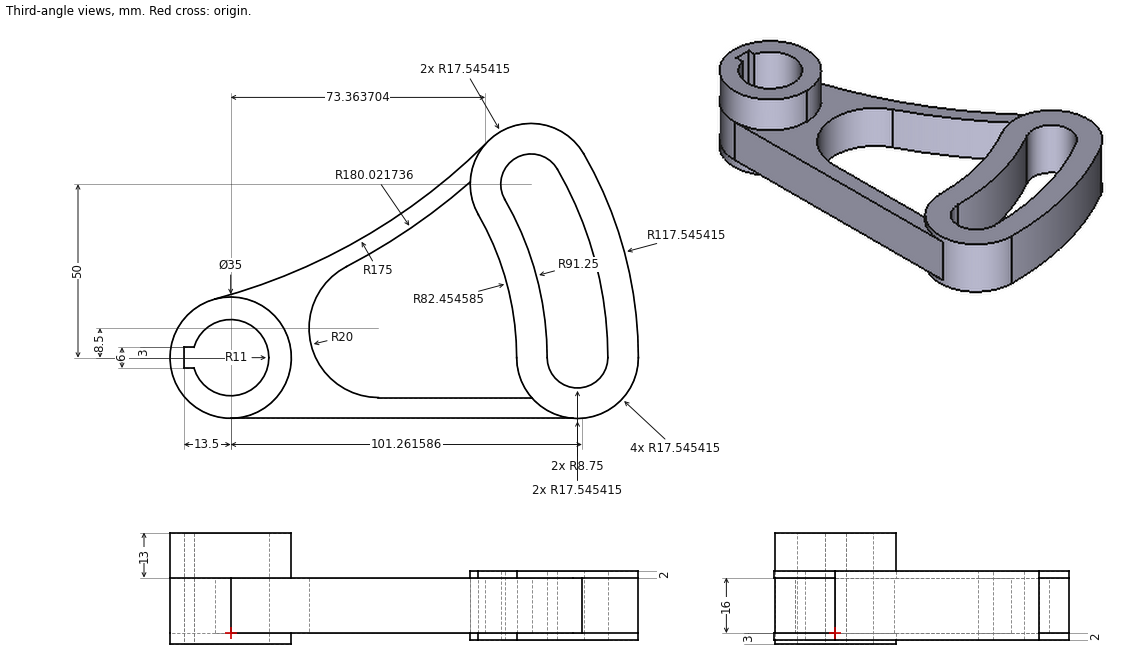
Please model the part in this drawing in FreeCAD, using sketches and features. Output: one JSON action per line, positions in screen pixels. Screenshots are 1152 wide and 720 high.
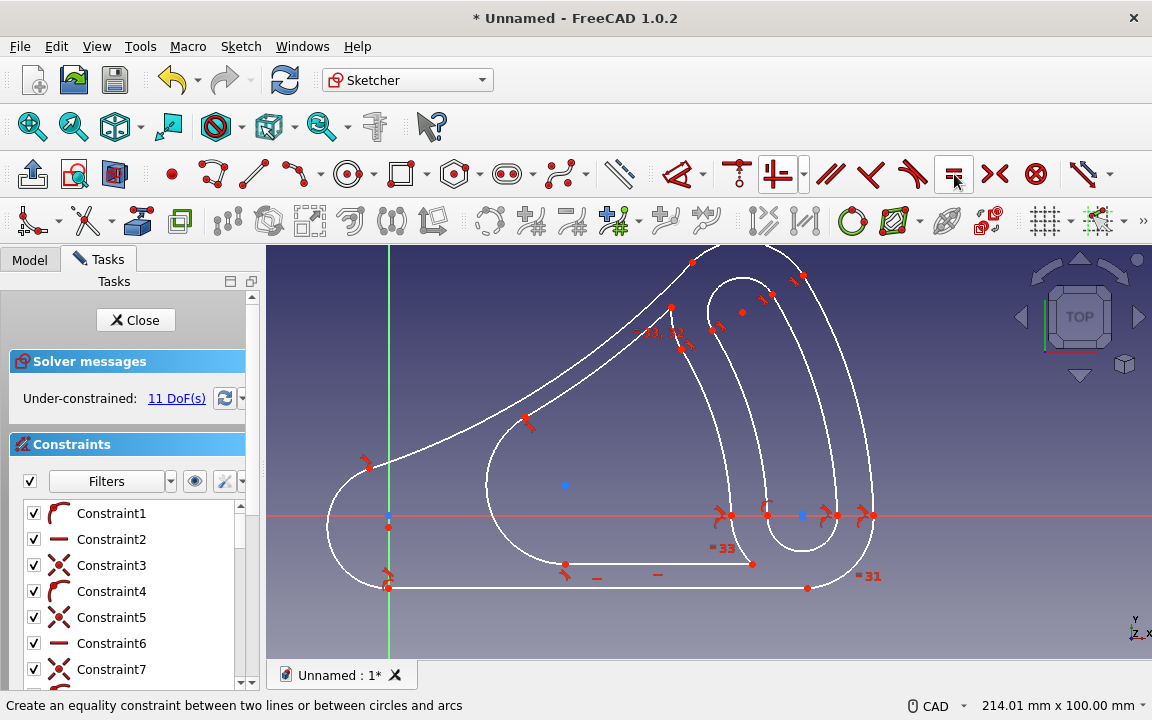
{"action": "left_click", "coordinate": [389, 527]}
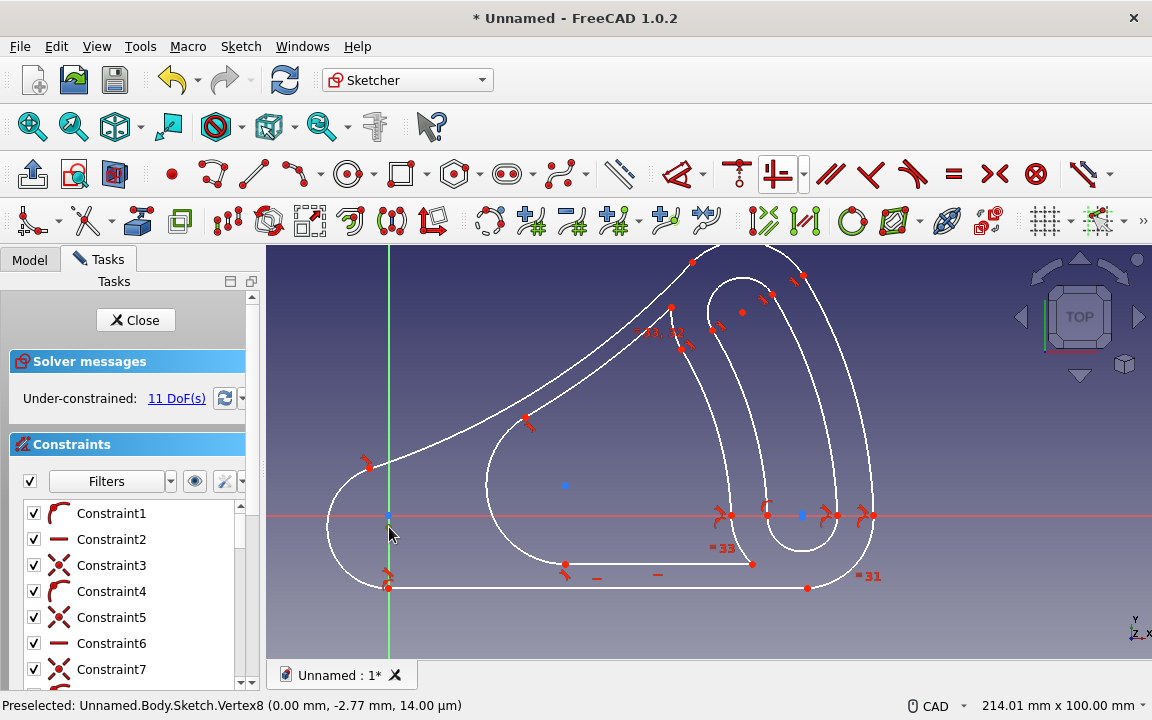
{"action": "left_click", "coordinate": [442, 516]}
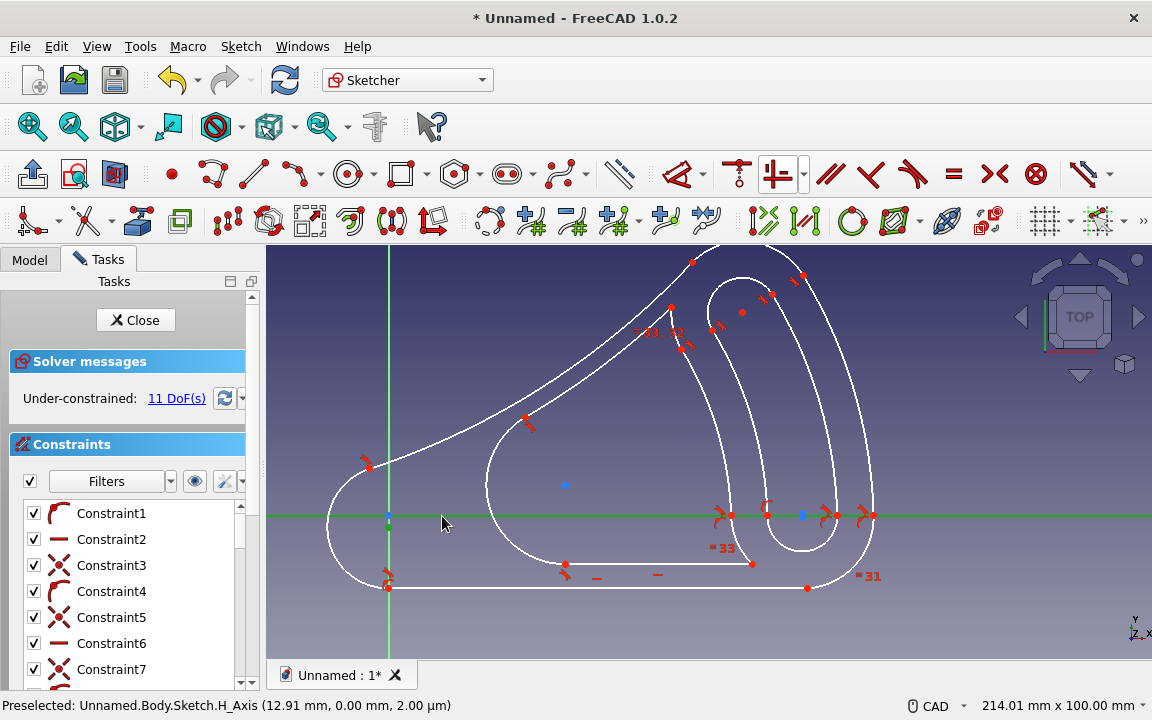
{"action": "left_click", "coordinate": [737, 174]}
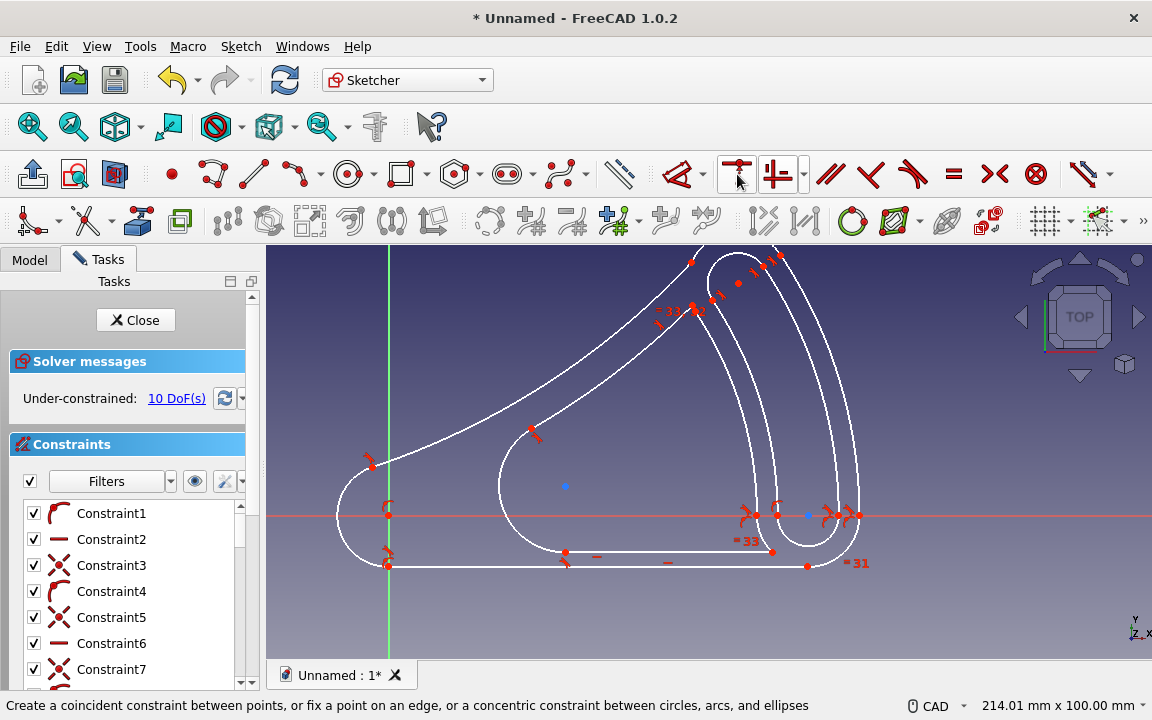
{"action": "left_click", "coordinate": [676, 174]}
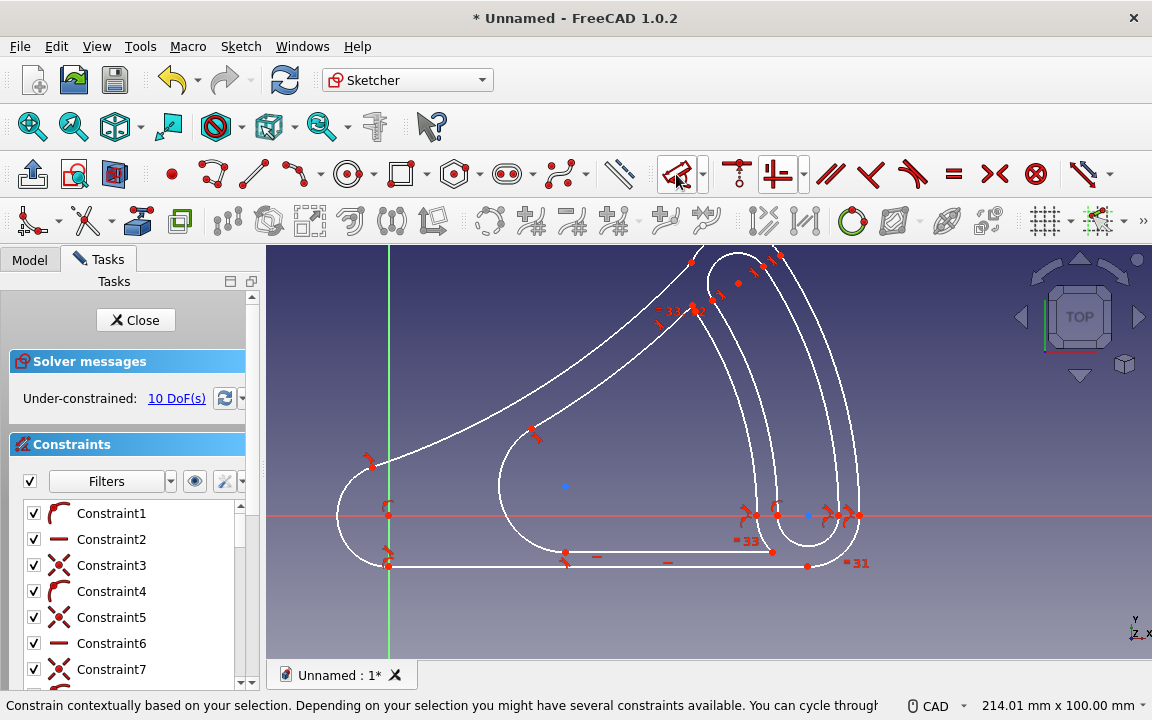
{"action": "left_click", "coordinate": [831, 562]}
{"action": "left_click", "coordinate": [845, 591]}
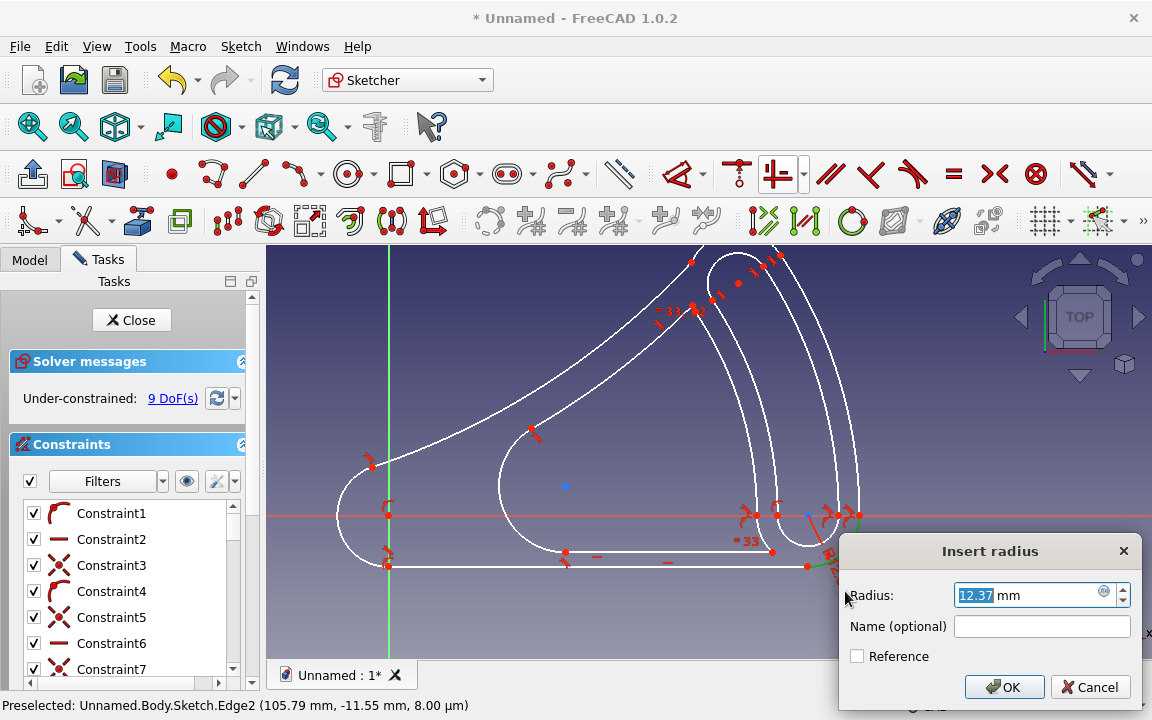
{"action": "type", "text": "17.545415"}
{"action": "key", "text": "Return"}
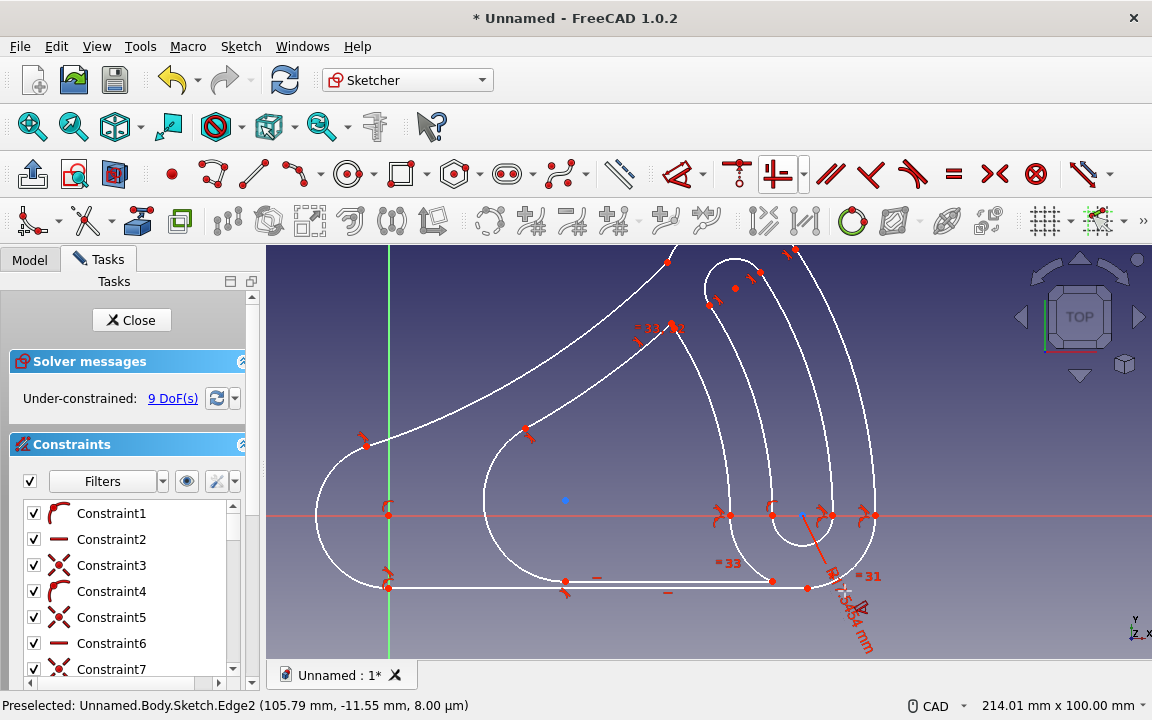
{"action": "left_click", "coordinate": [868, 432]}
{"action": "left_click", "coordinate": [900, 426]}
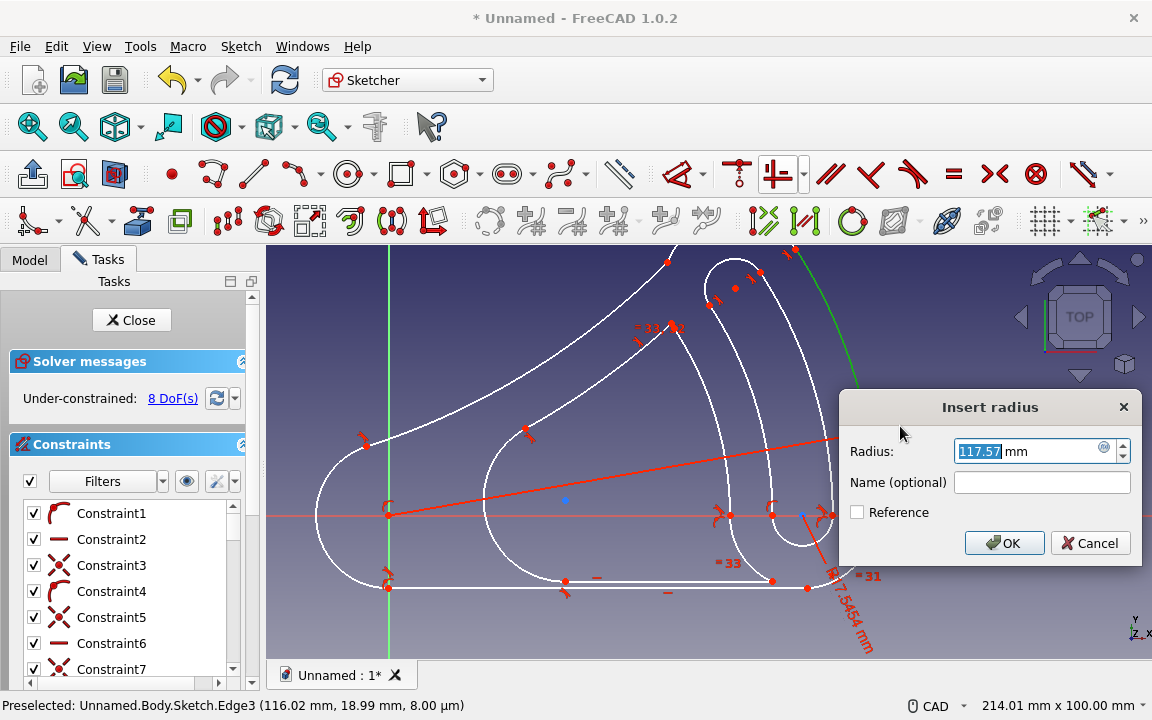
{"action": "type", "text": "117.545415"}
{"action": "key", "text": "Return"}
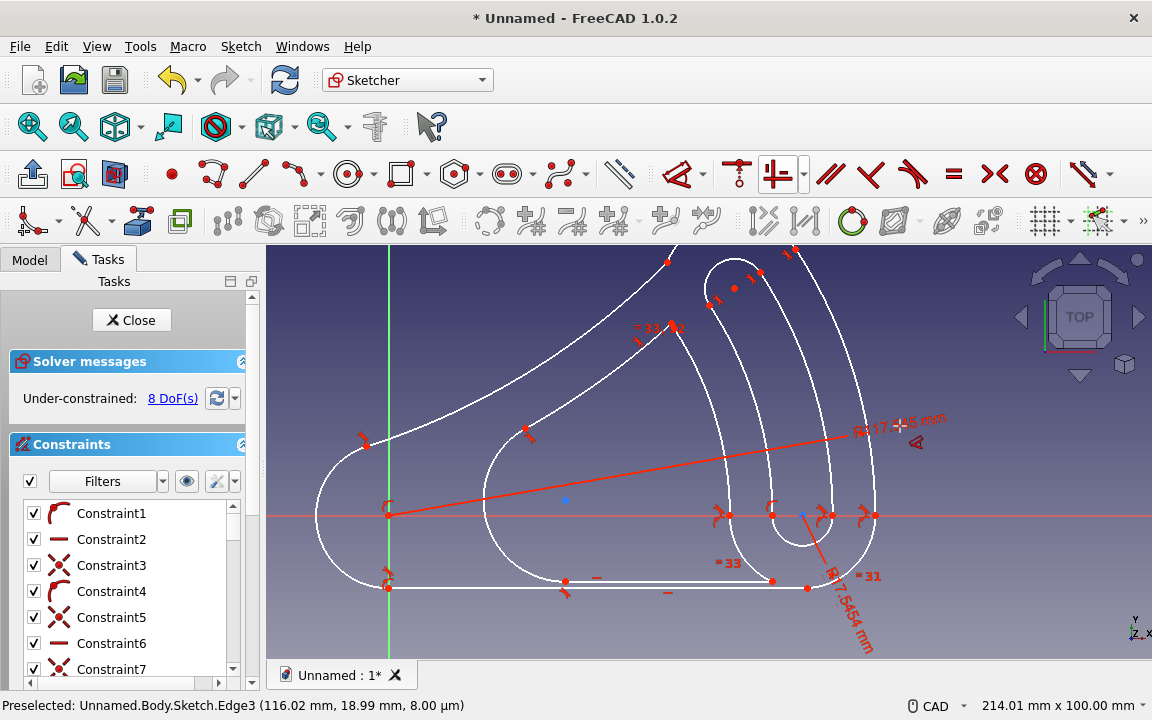
{"action": "left_click", "coordinate": [466, 407]}
{"action": "left_click", "coordinate": [480, 436]}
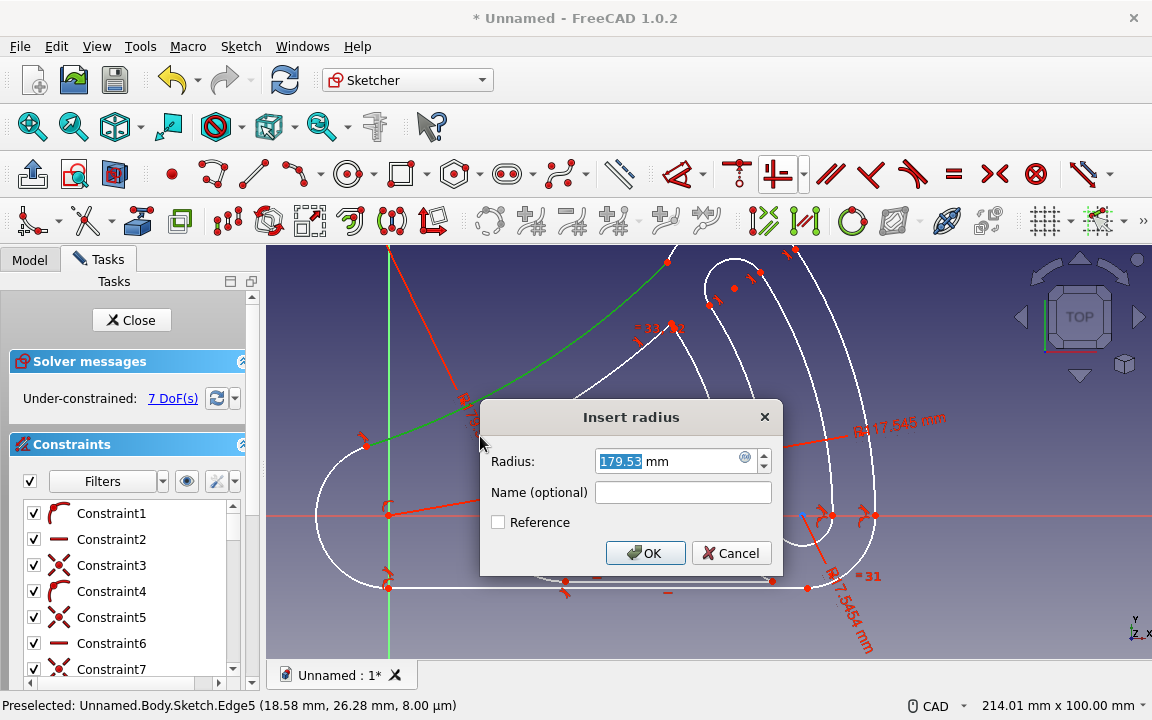
{"action": "type", "text": "175"}
{"action": "key", "text": "Return"}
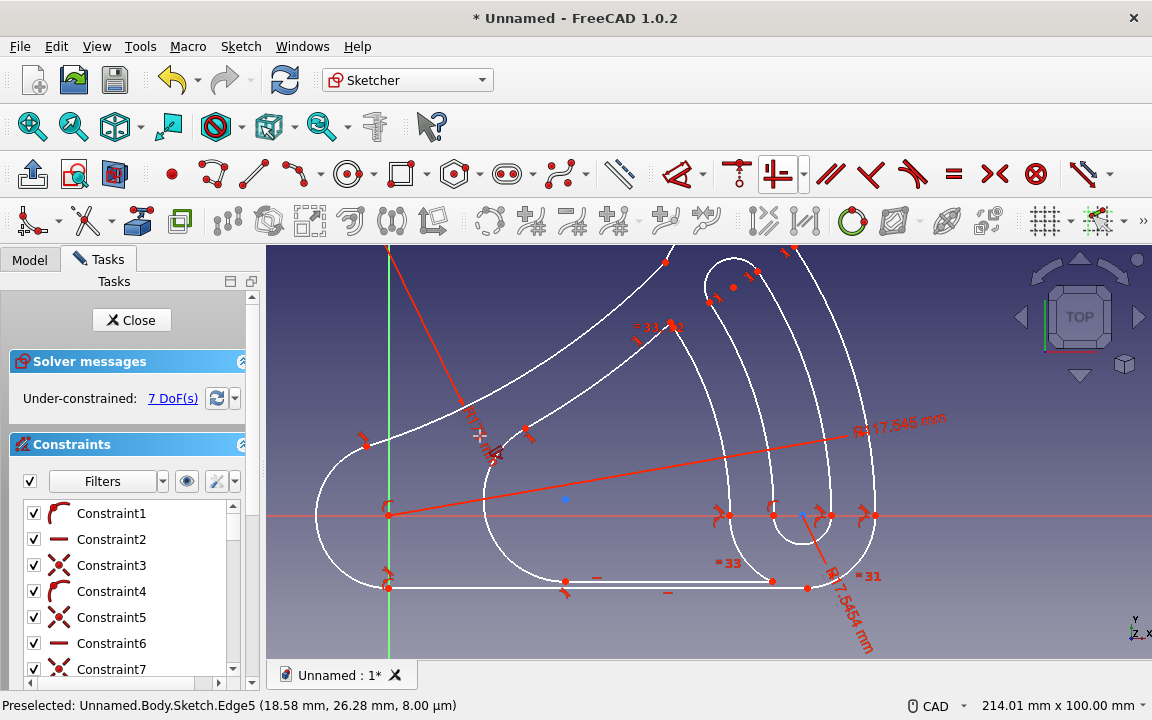
{"action": "left_click", "coordinate": [486, 478]}
{"action": "left_click", "coordinate": [455, 469]}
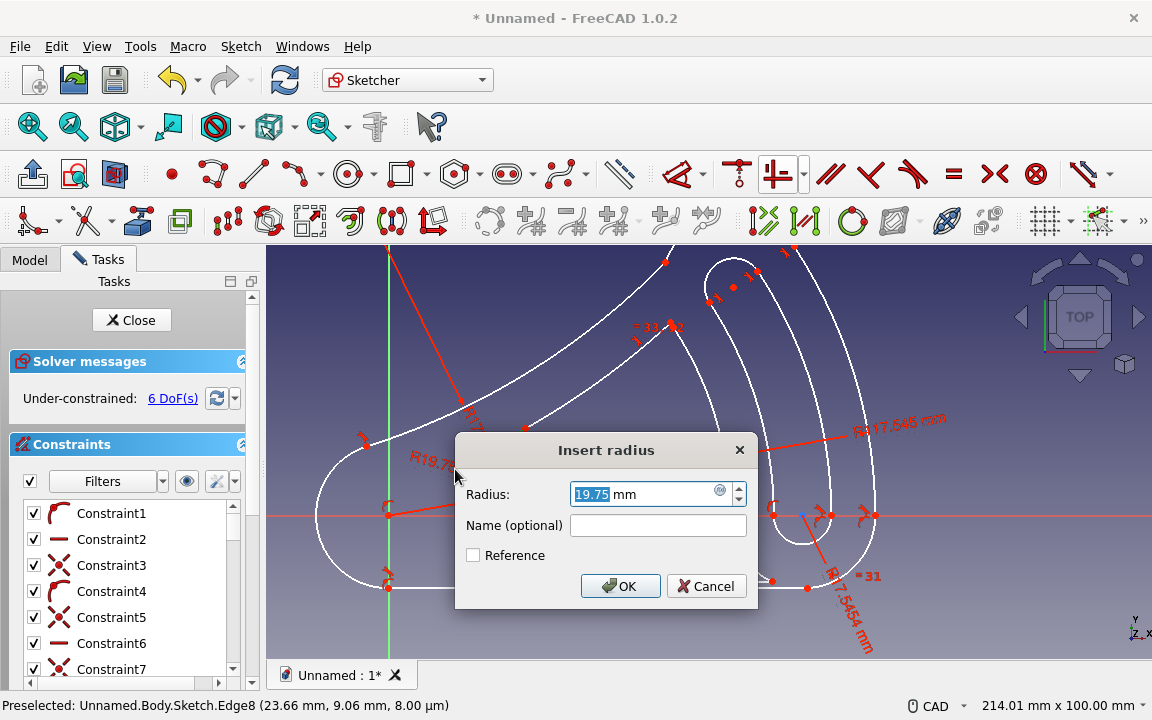
{"action": "type", "text": "20"}
{"action": "key", "text": "Return"}